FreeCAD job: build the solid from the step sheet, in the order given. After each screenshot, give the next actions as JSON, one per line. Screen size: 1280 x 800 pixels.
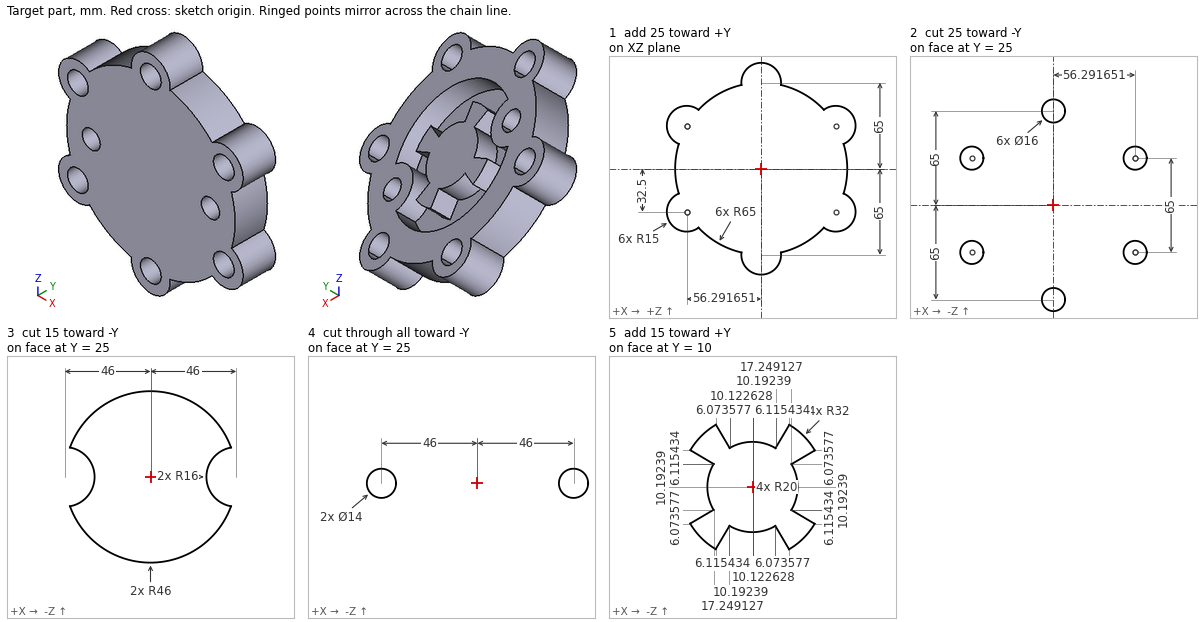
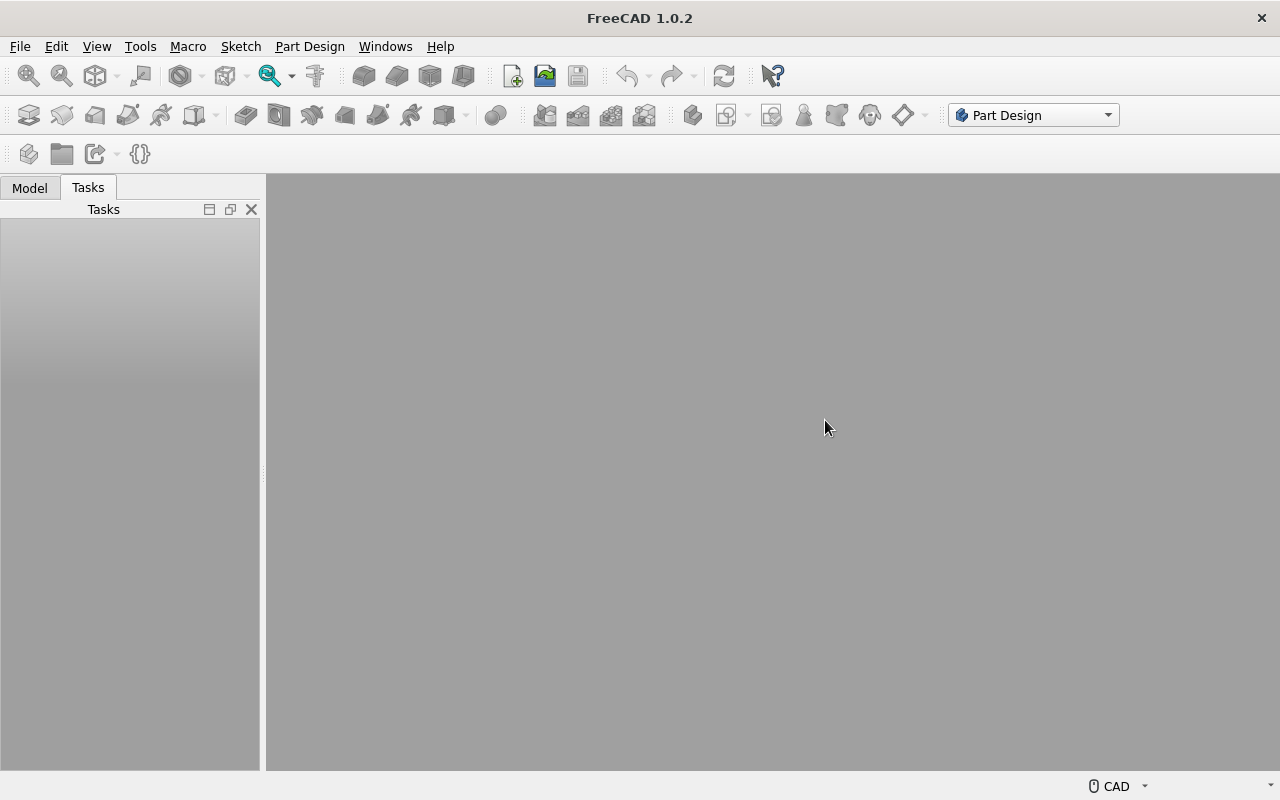
{"action": "left_click", "coordinate": [512, 76]}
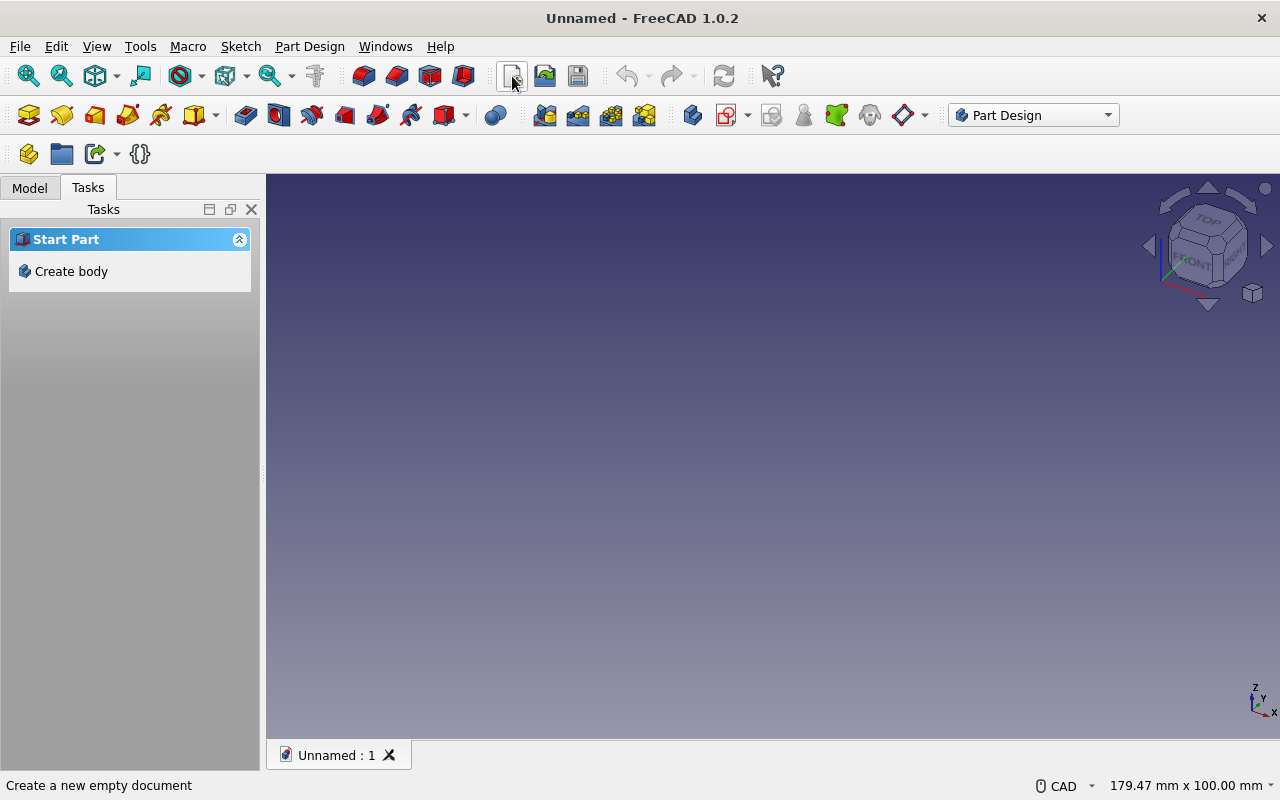
{"action": "left_click", "coordinate": [726, 116]}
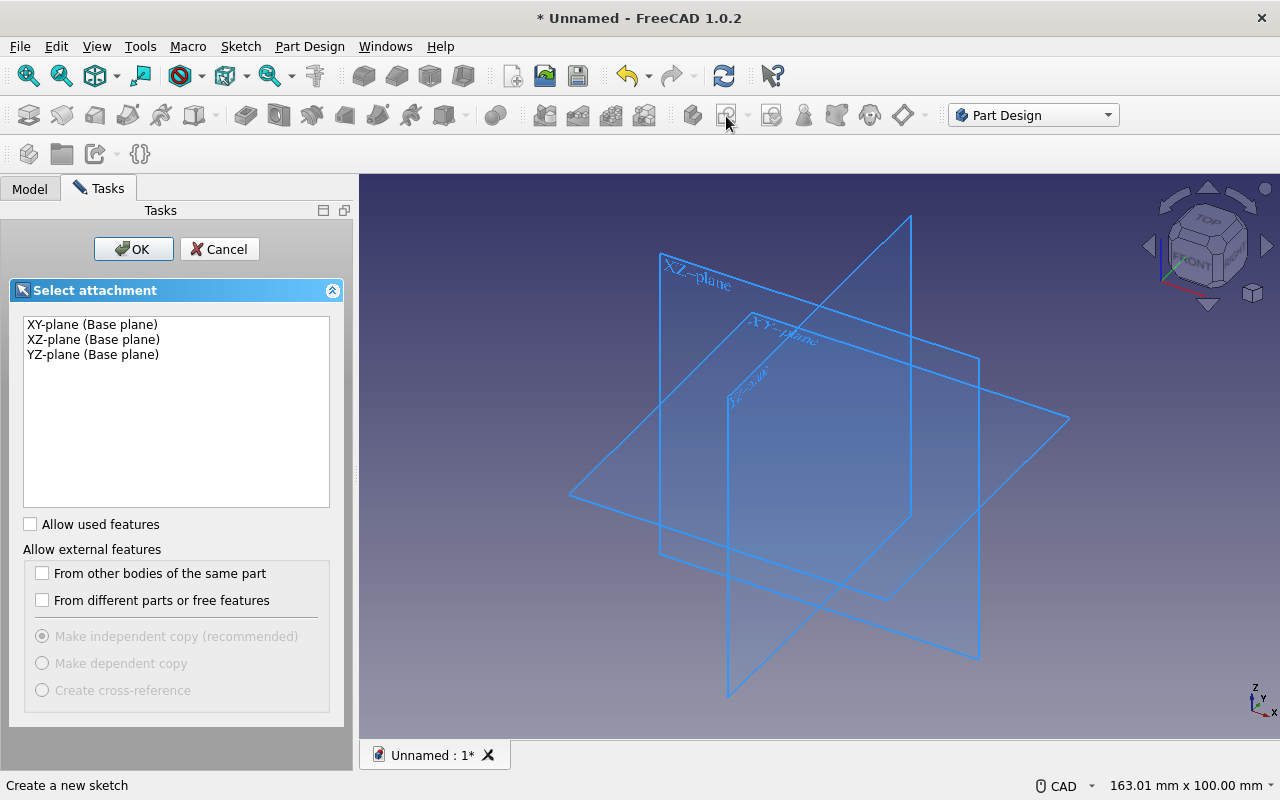
{"action": "left_click", "coordinate": [84, 340]}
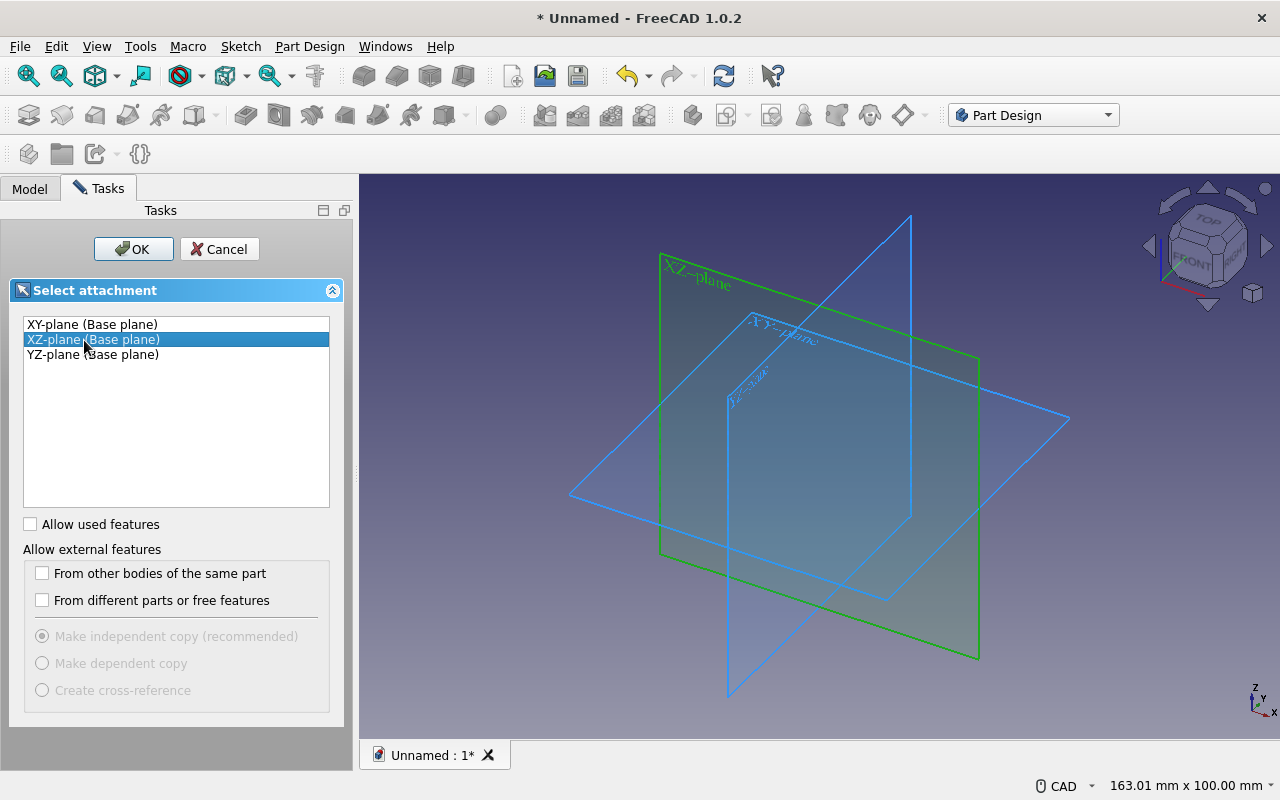
{"action": "left_click", "coordinate": [134, 249]}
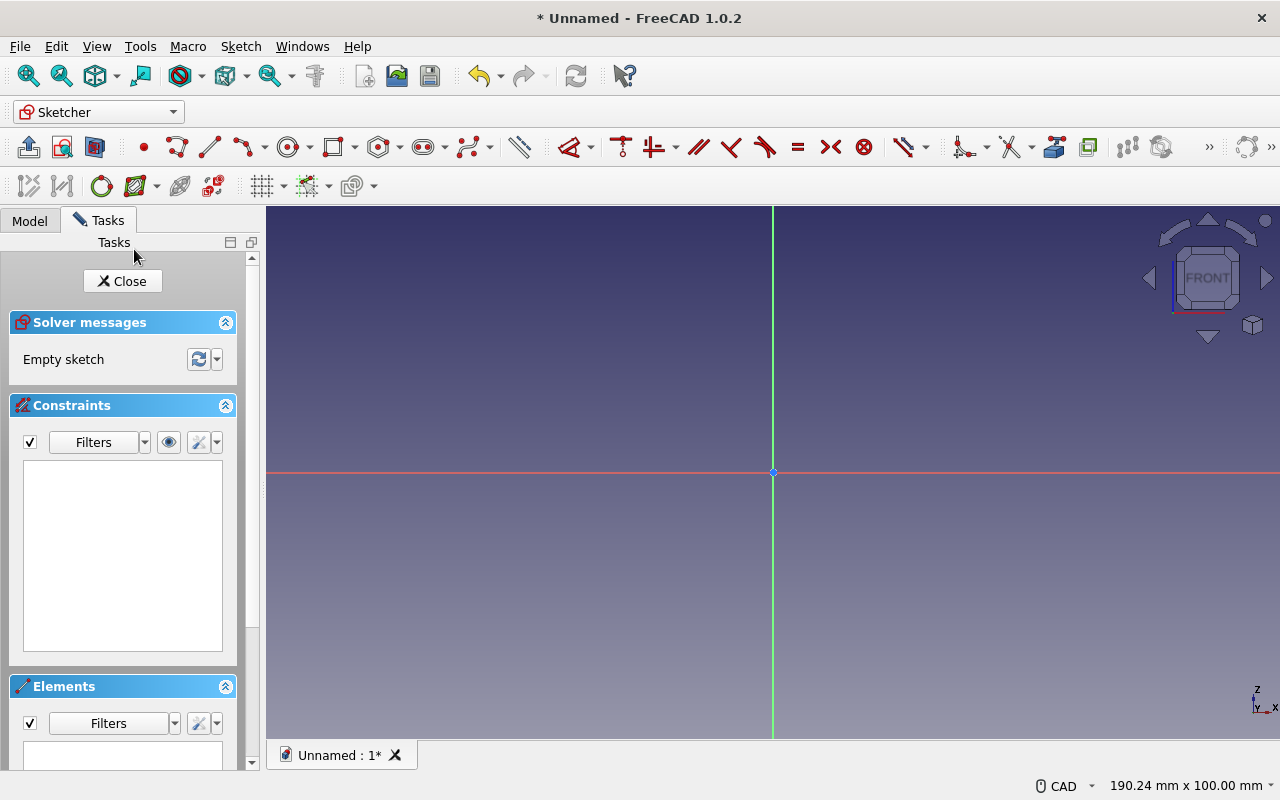
{"action": "scroll", "coordinate": [665, 472], "scroll_direction": "down", "scroll_amount": 5}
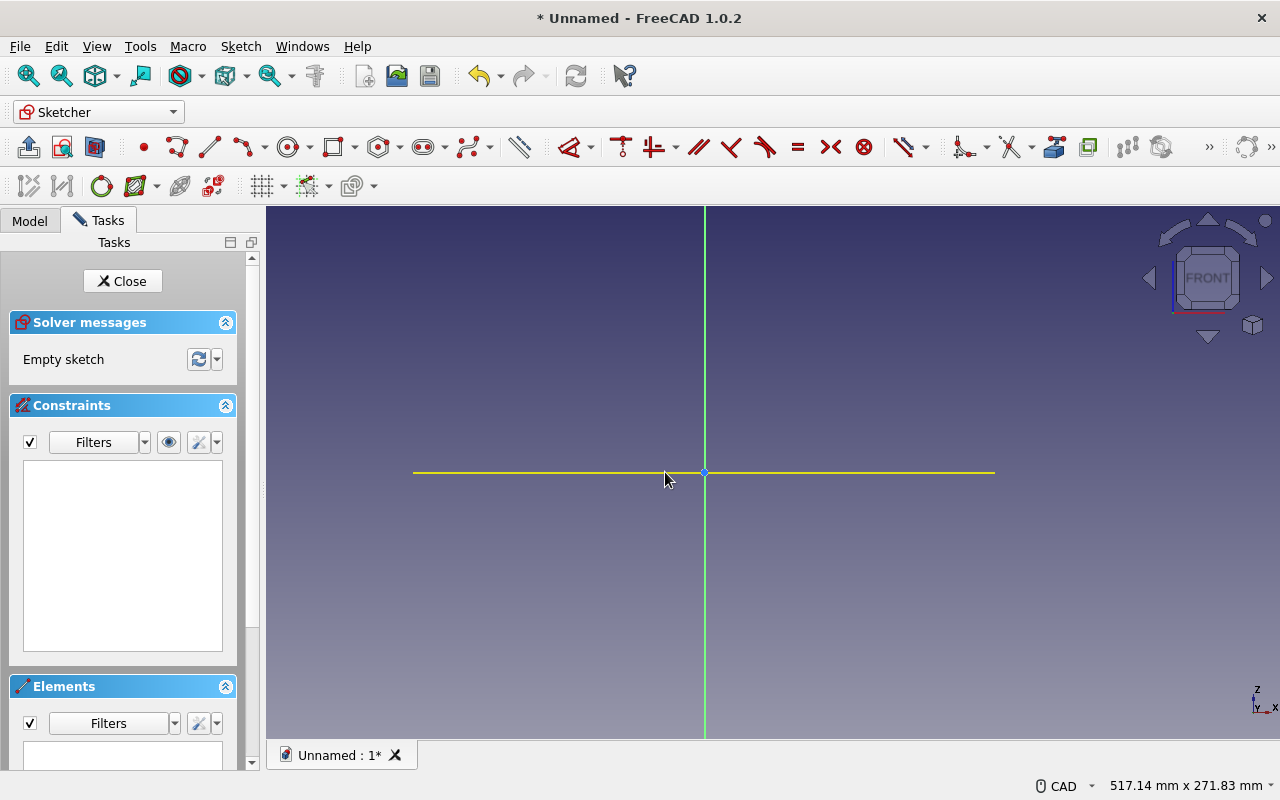
{"action": "left_click", "coordinate": [242, 148]}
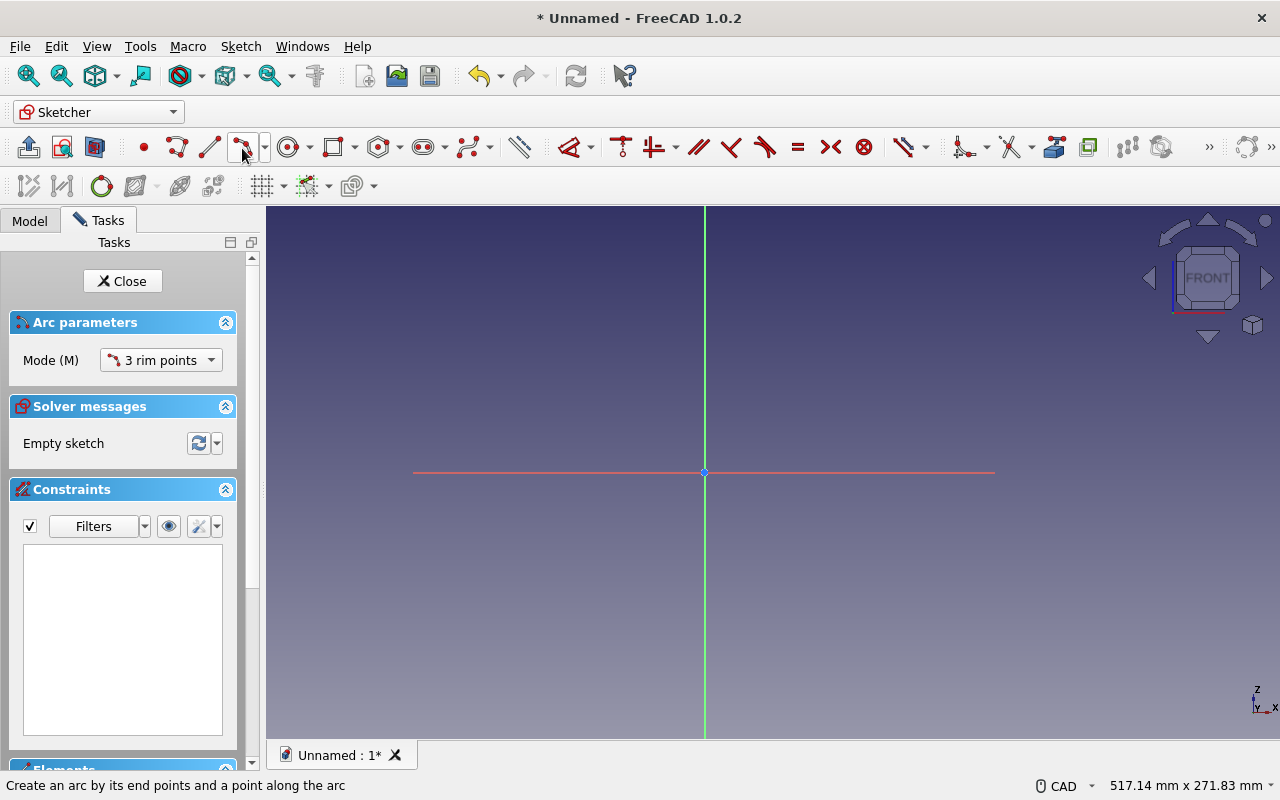
{"action": "left_click", "coordinate": [676, 597]}
{"action": "left_click", "coordinate": [612, 560]}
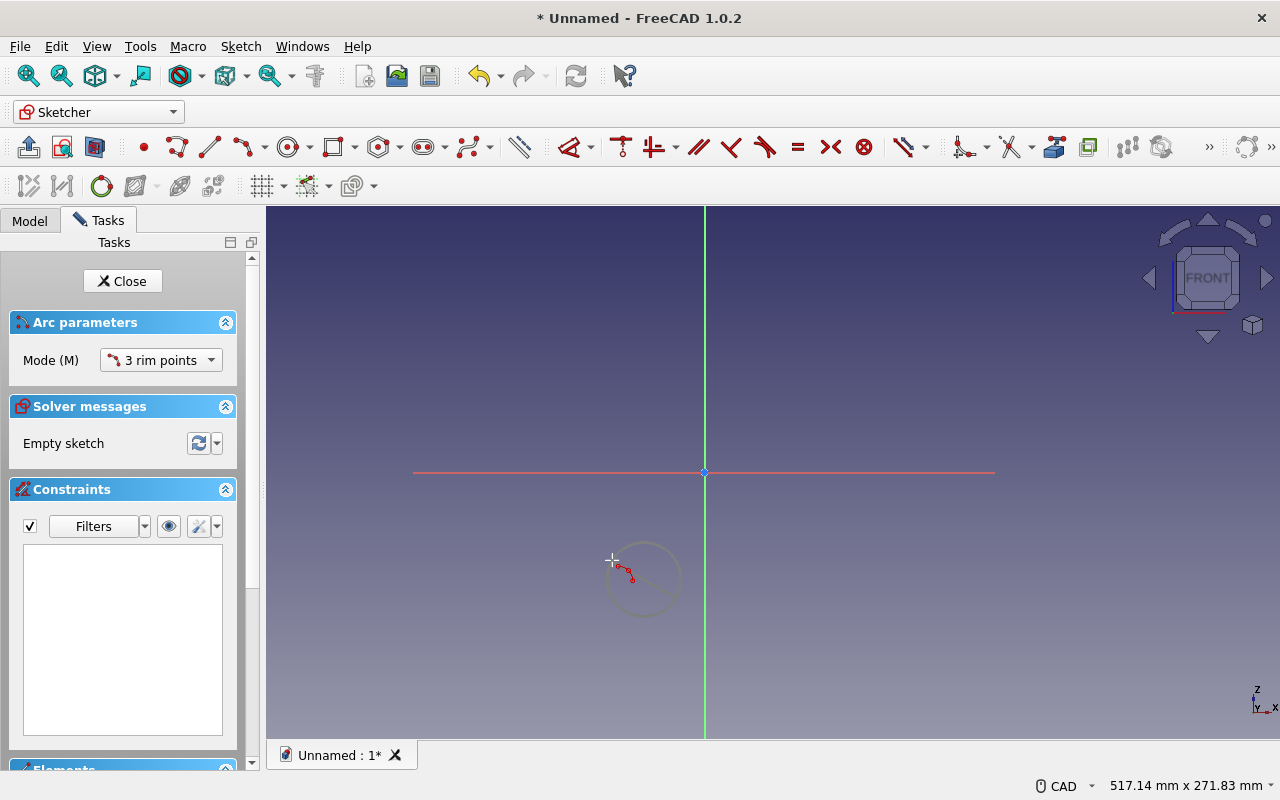
{"action": "scroll", "coordinate": [641, 583], "scroll_direction": "up", "scroll_amount": 6}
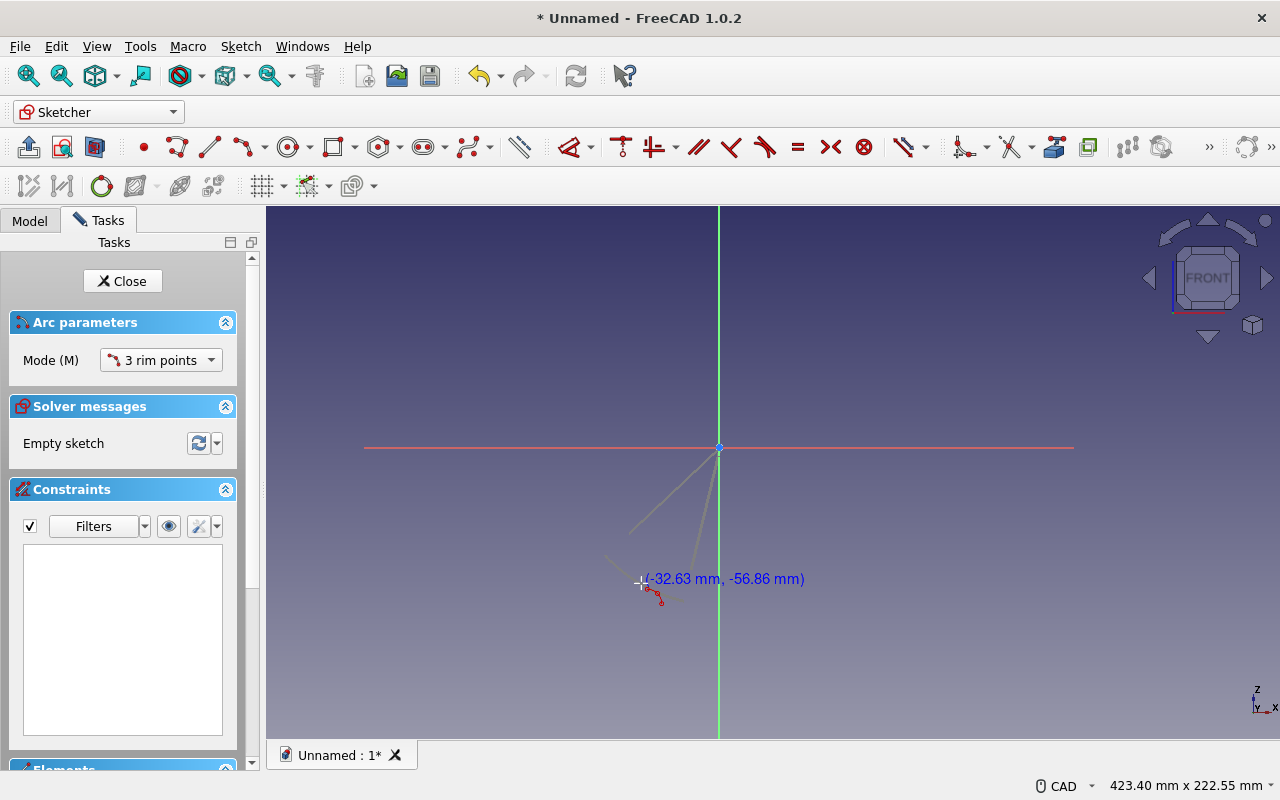
{"action": "left_click", "coordinate": [641, 581]}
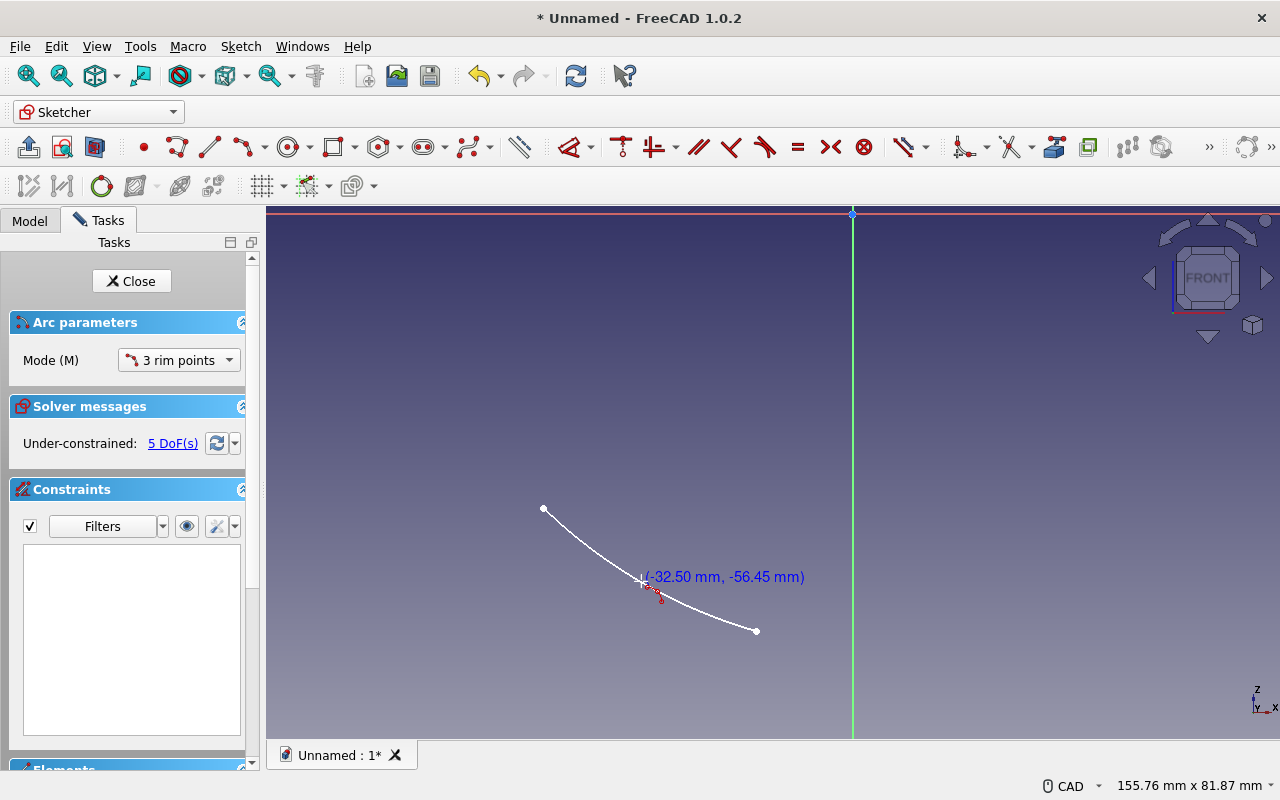
{"action": "left_click", "coordinate": [544, 508]}
{"action": "left_click", "coordinate": [447, 336]}
{"action": "left_click", "coordinate": [402, 475]}